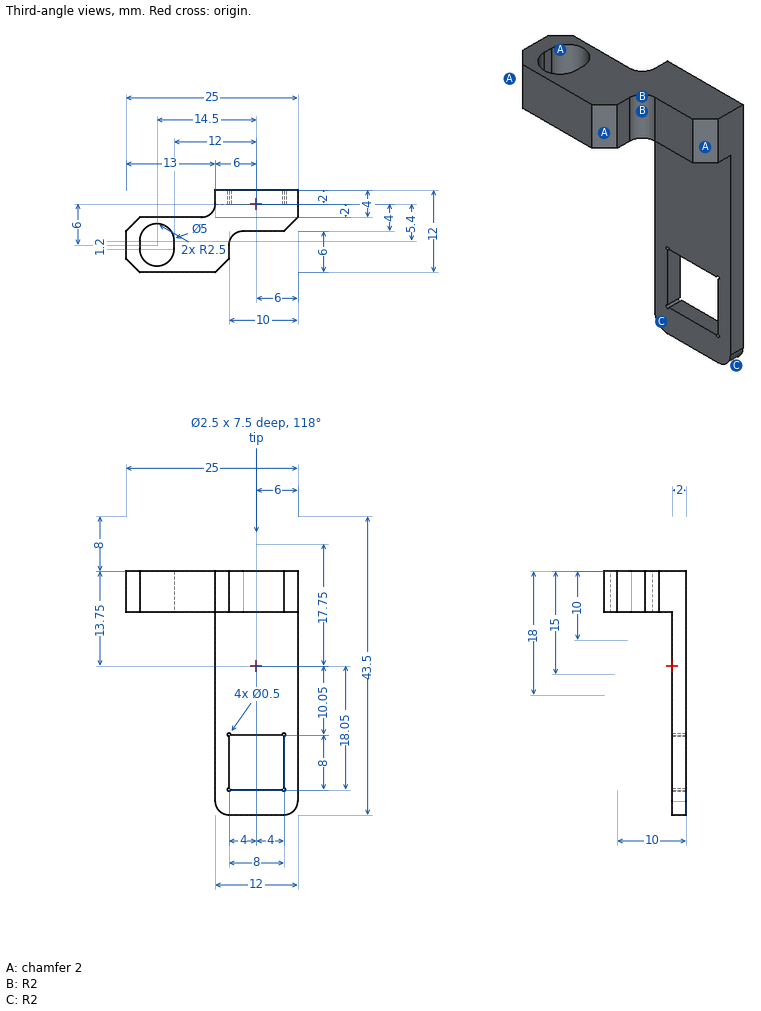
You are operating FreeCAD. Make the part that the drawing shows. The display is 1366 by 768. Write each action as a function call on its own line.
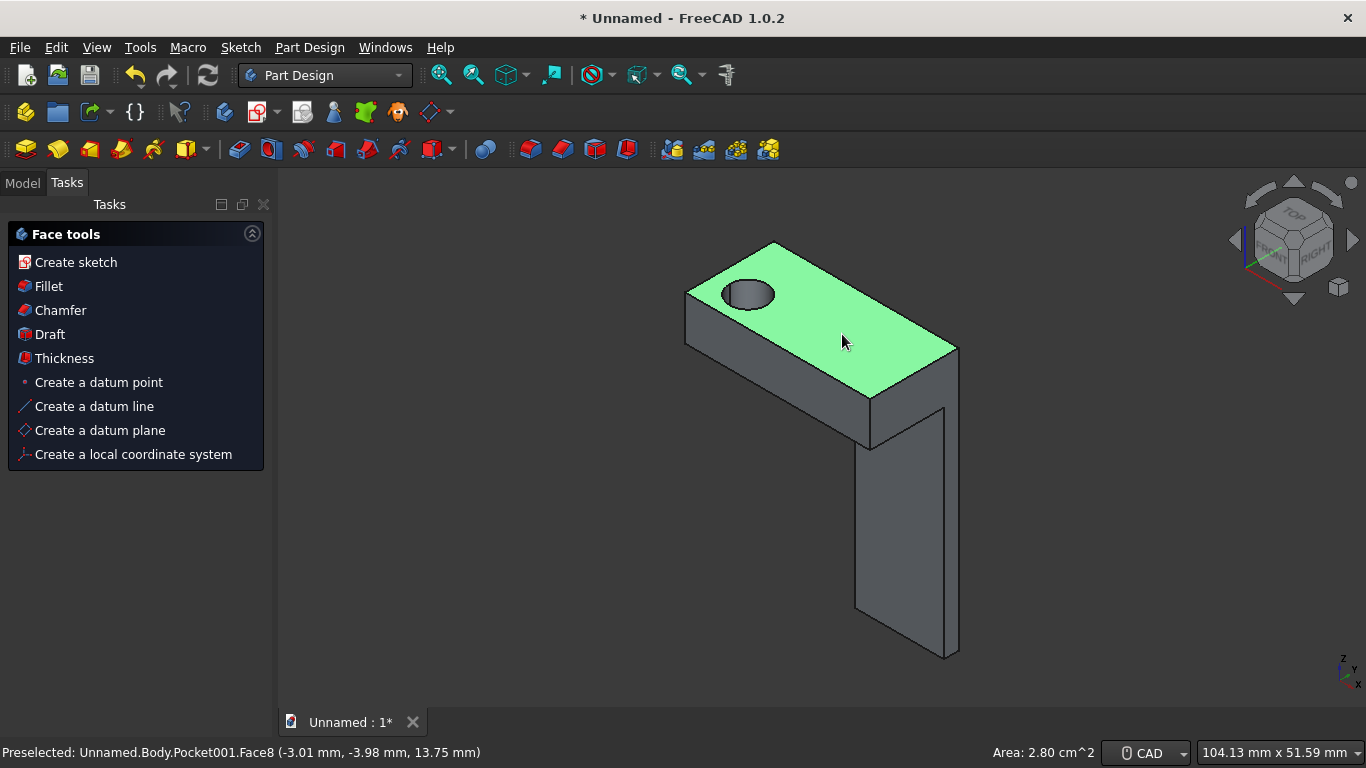
click(258, 112)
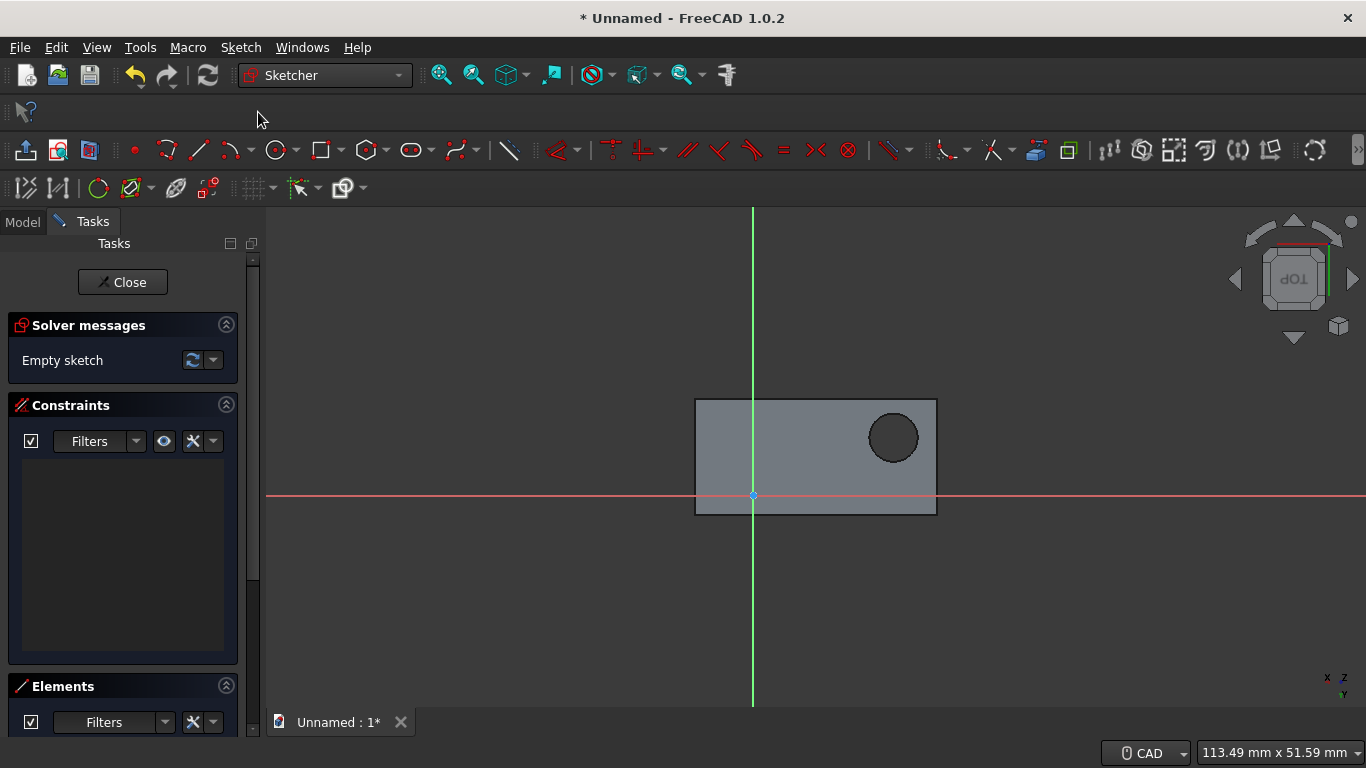
scroll(856, 457, up, 5)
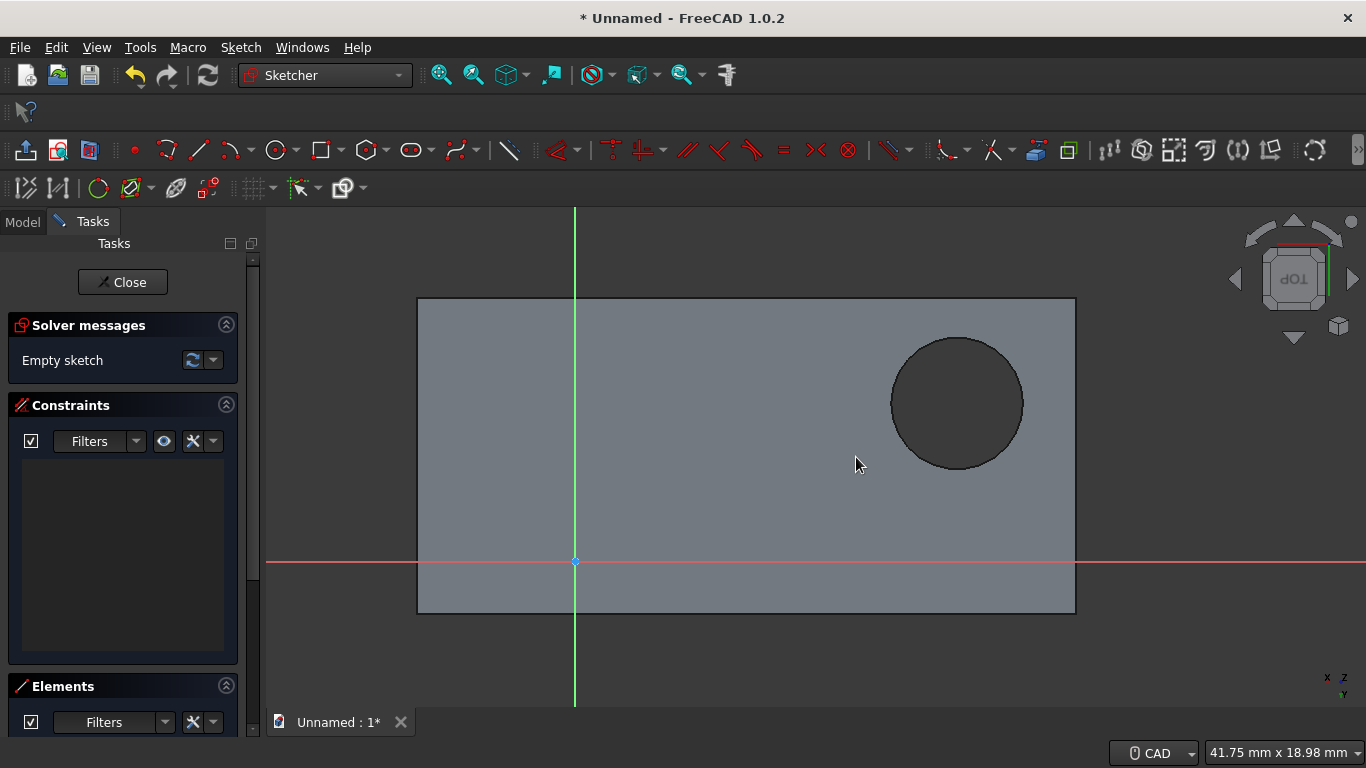
click(322, 150)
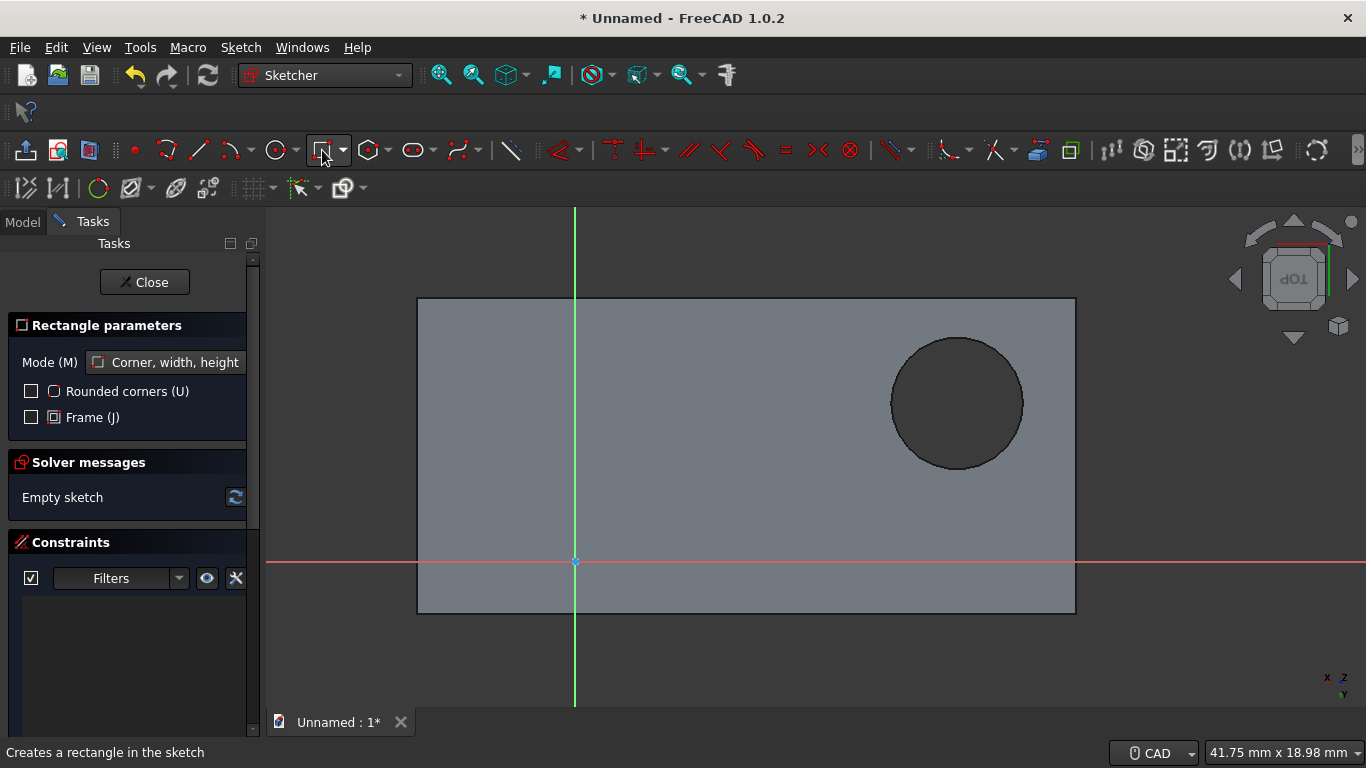
click(733, 509)
click(1076, 614)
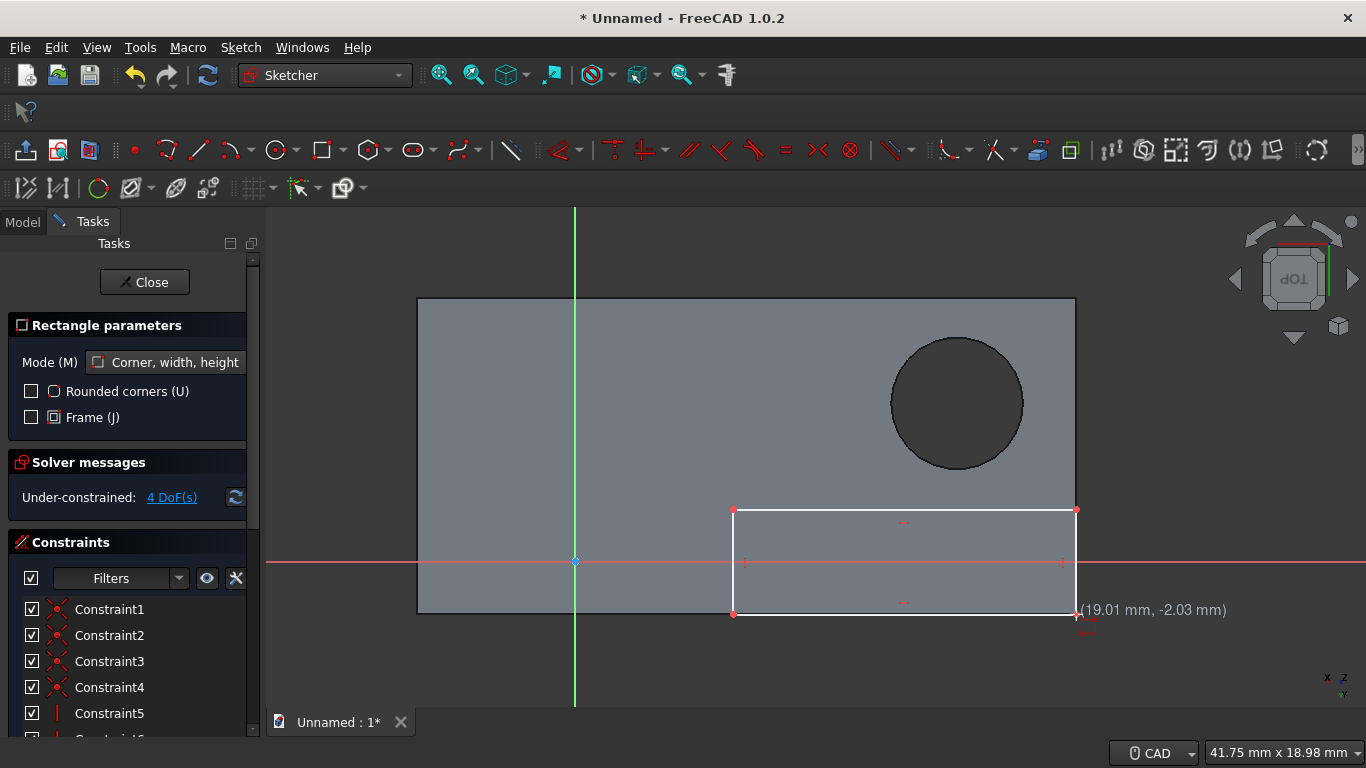
click(417, 298)
click(680, 456)
key(Escape)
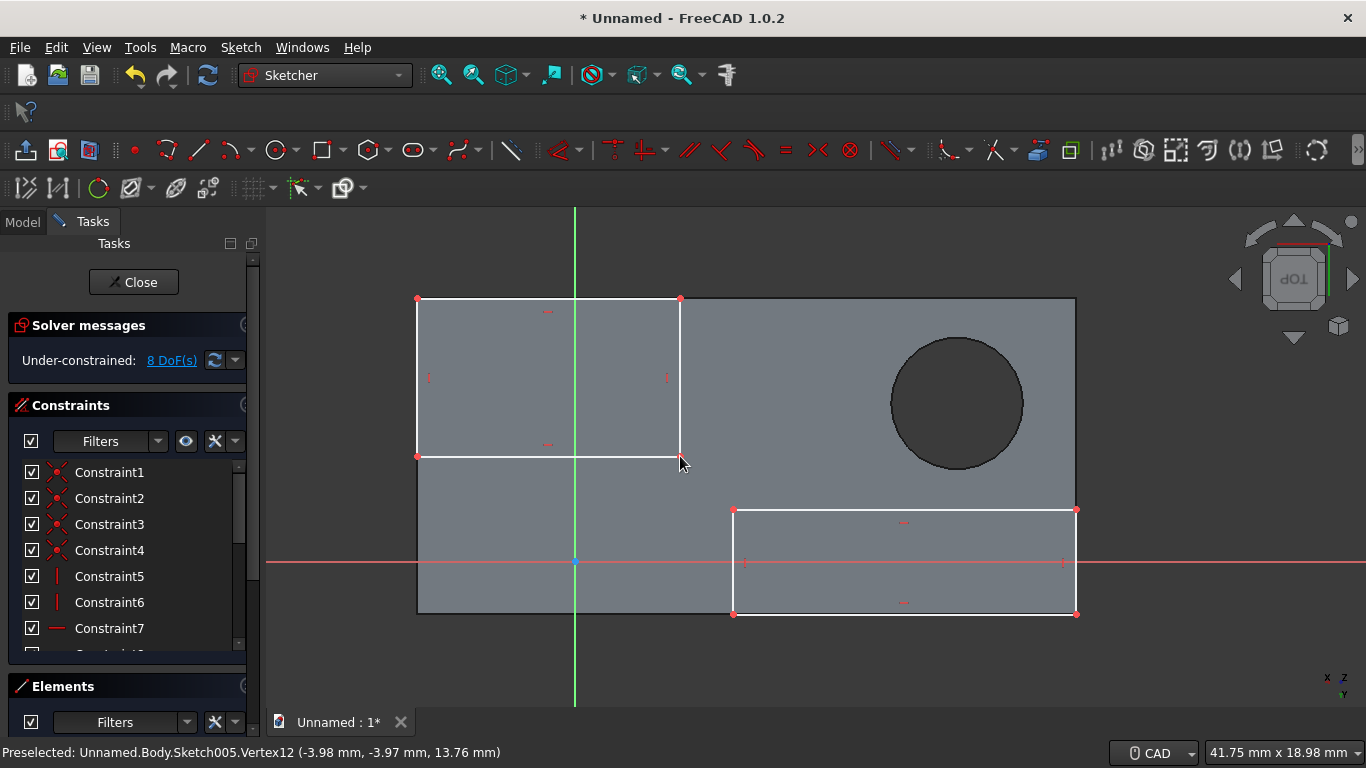
click(558, 150)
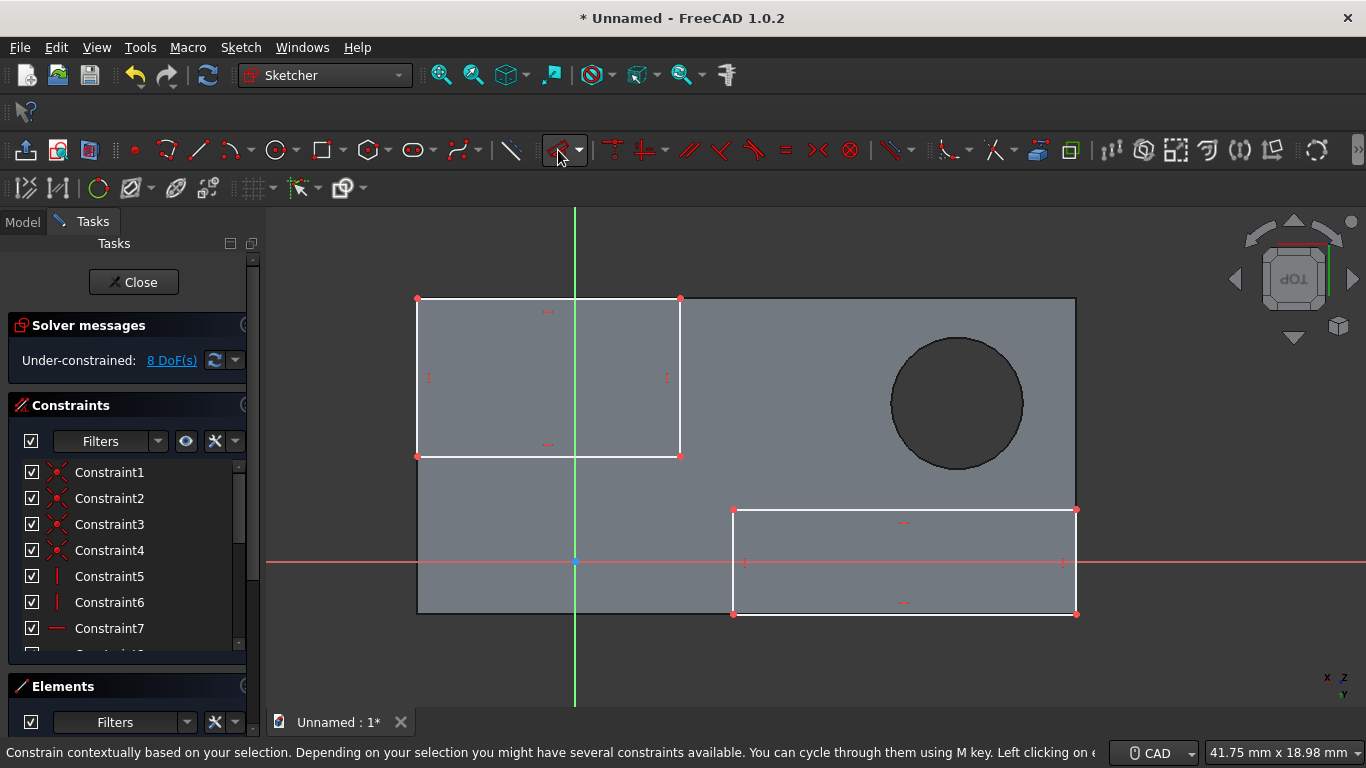
click(733, 541)
click(699, 538)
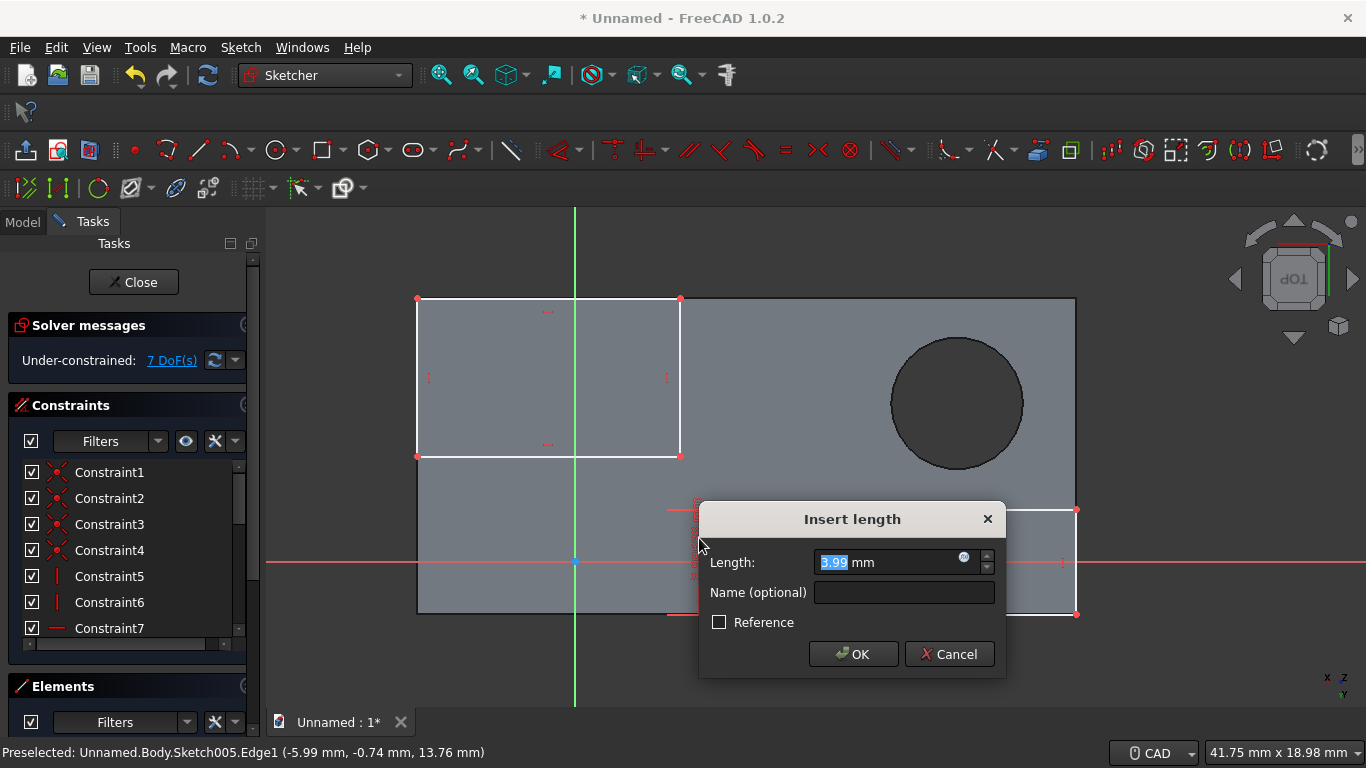
text(4)
key(Return)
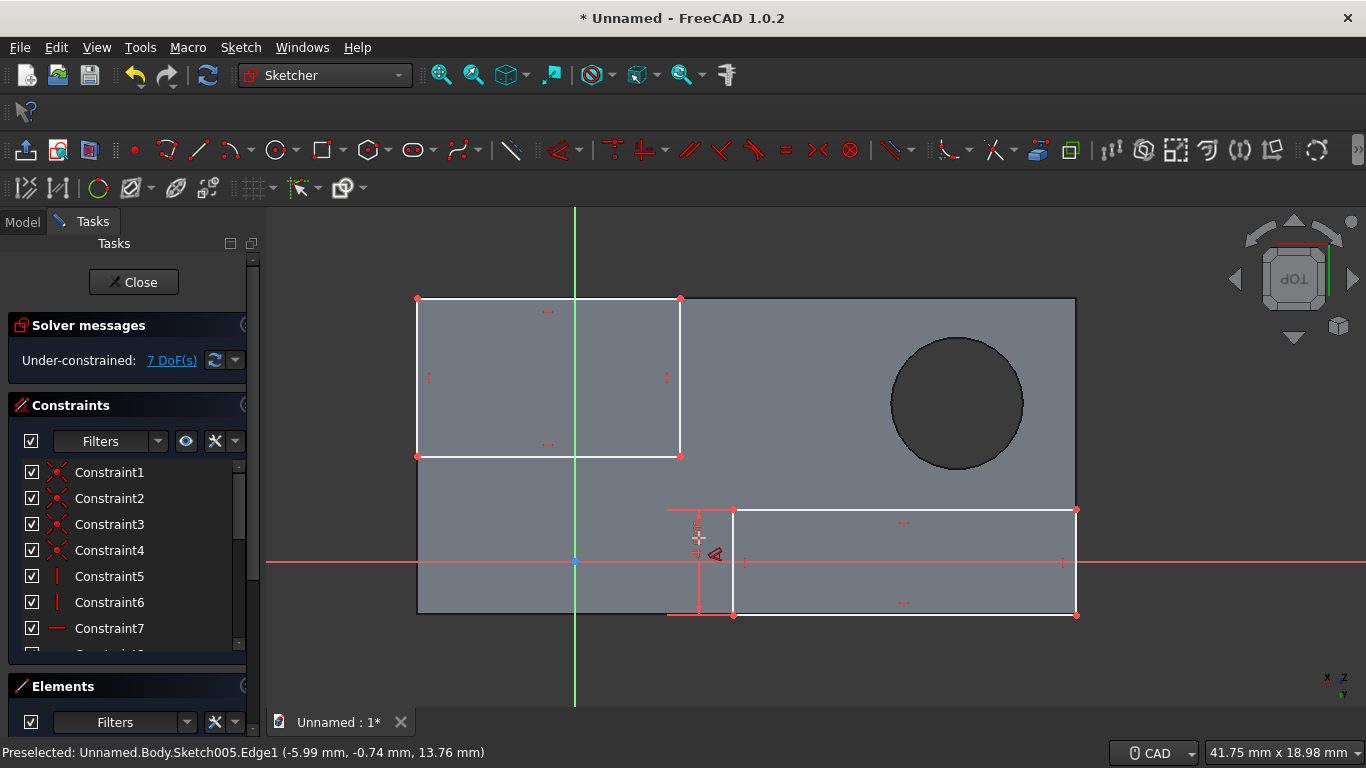
click(417, 346)
click(383, 378)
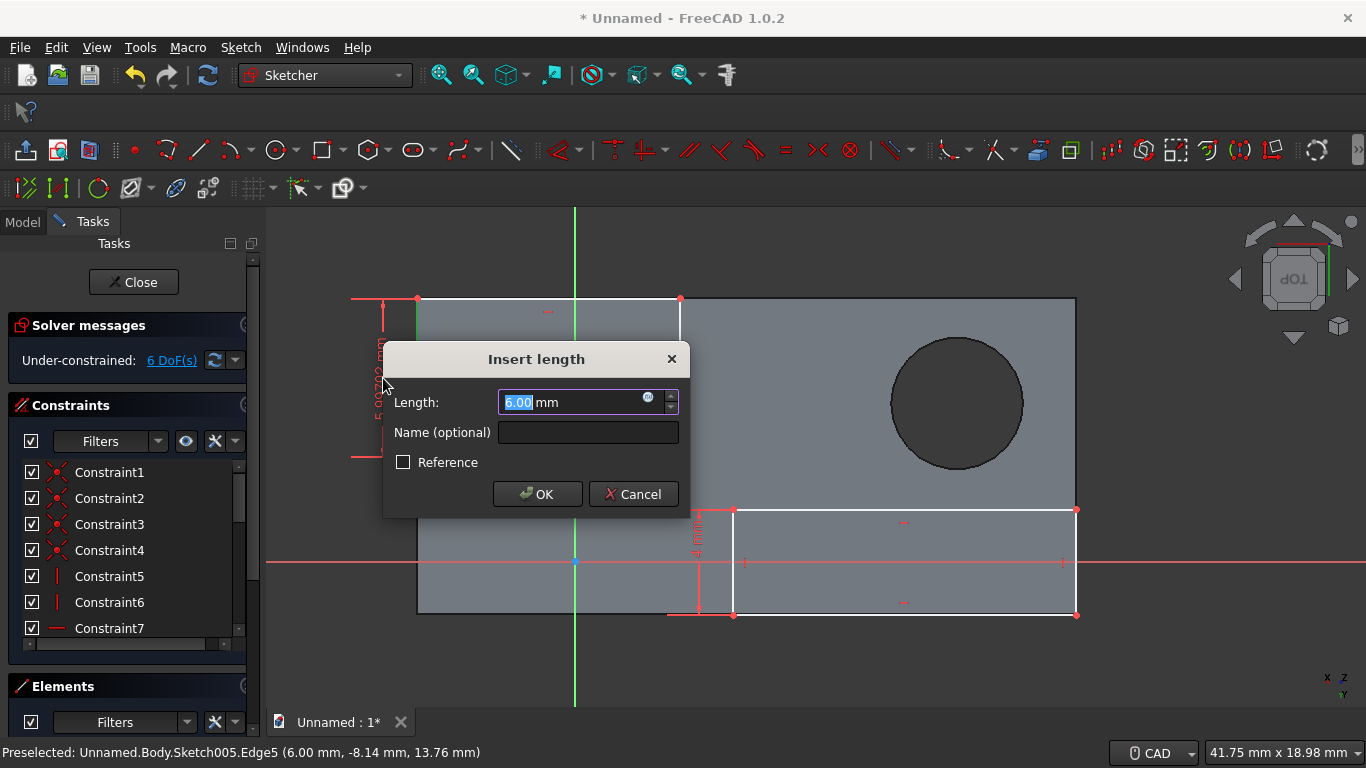
text(6)
key(Return)